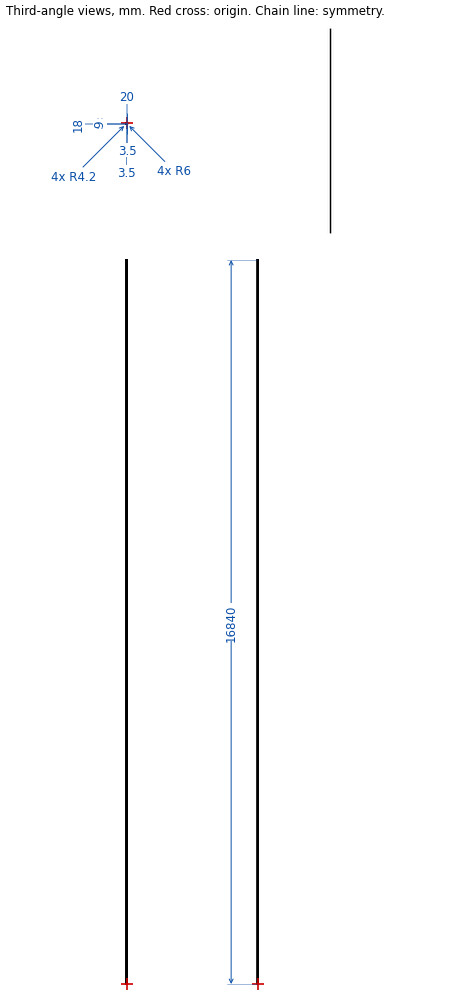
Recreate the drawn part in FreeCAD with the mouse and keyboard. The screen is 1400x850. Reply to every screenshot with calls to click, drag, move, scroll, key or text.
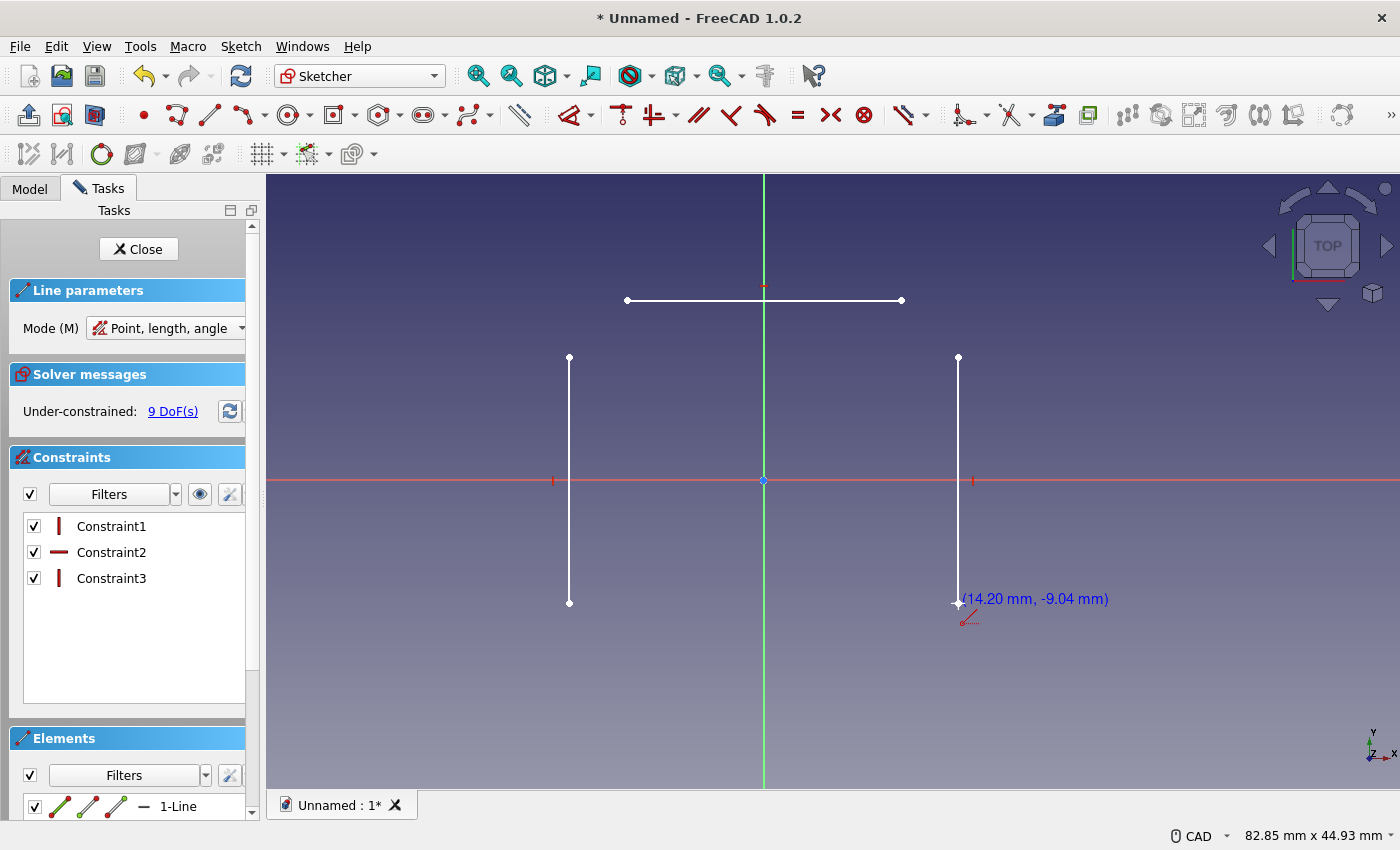
click(177, 116)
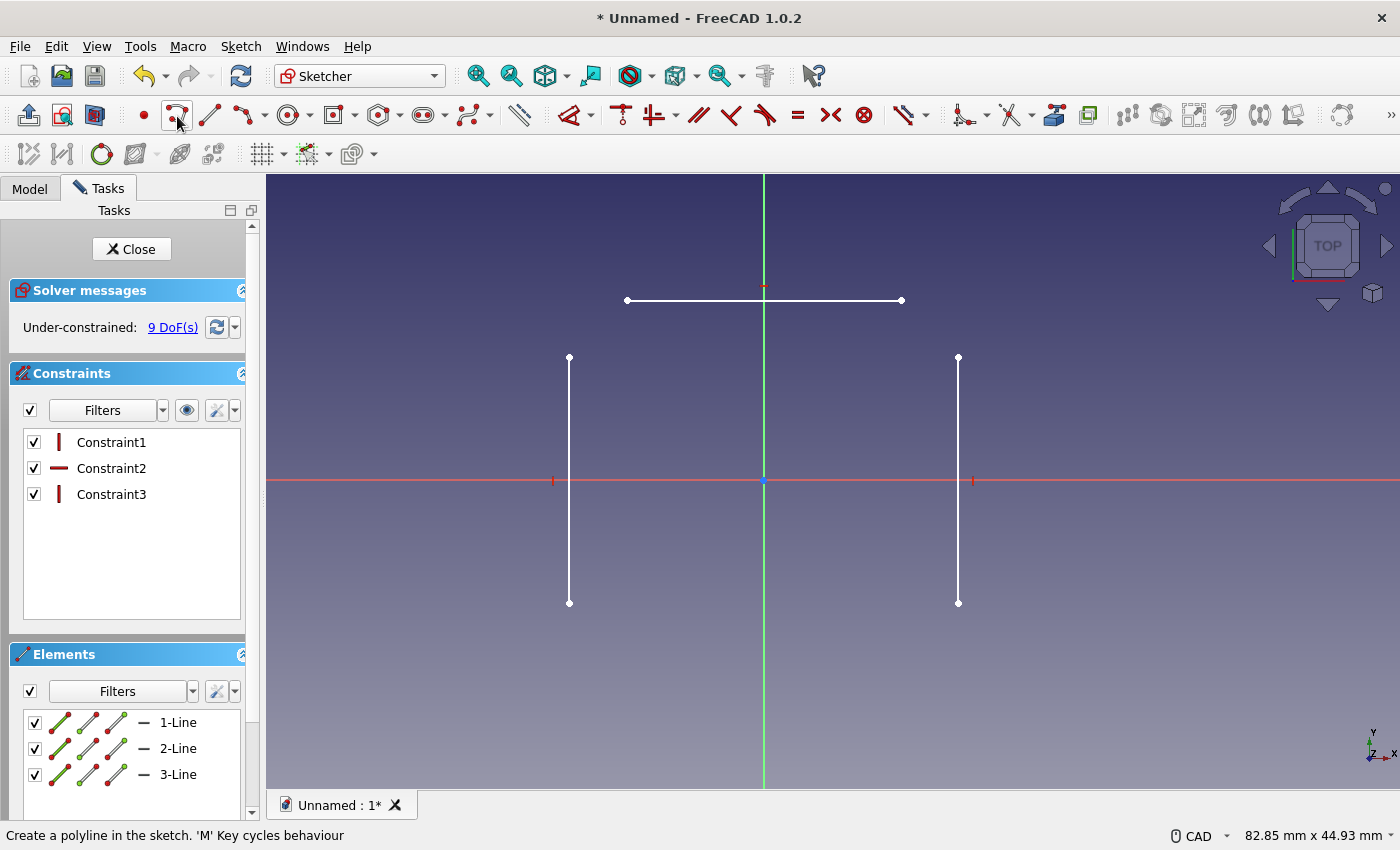
click(901, 661)
click(853, 661)
click(853, 686)
click(901, 686)
right_click(901, 686)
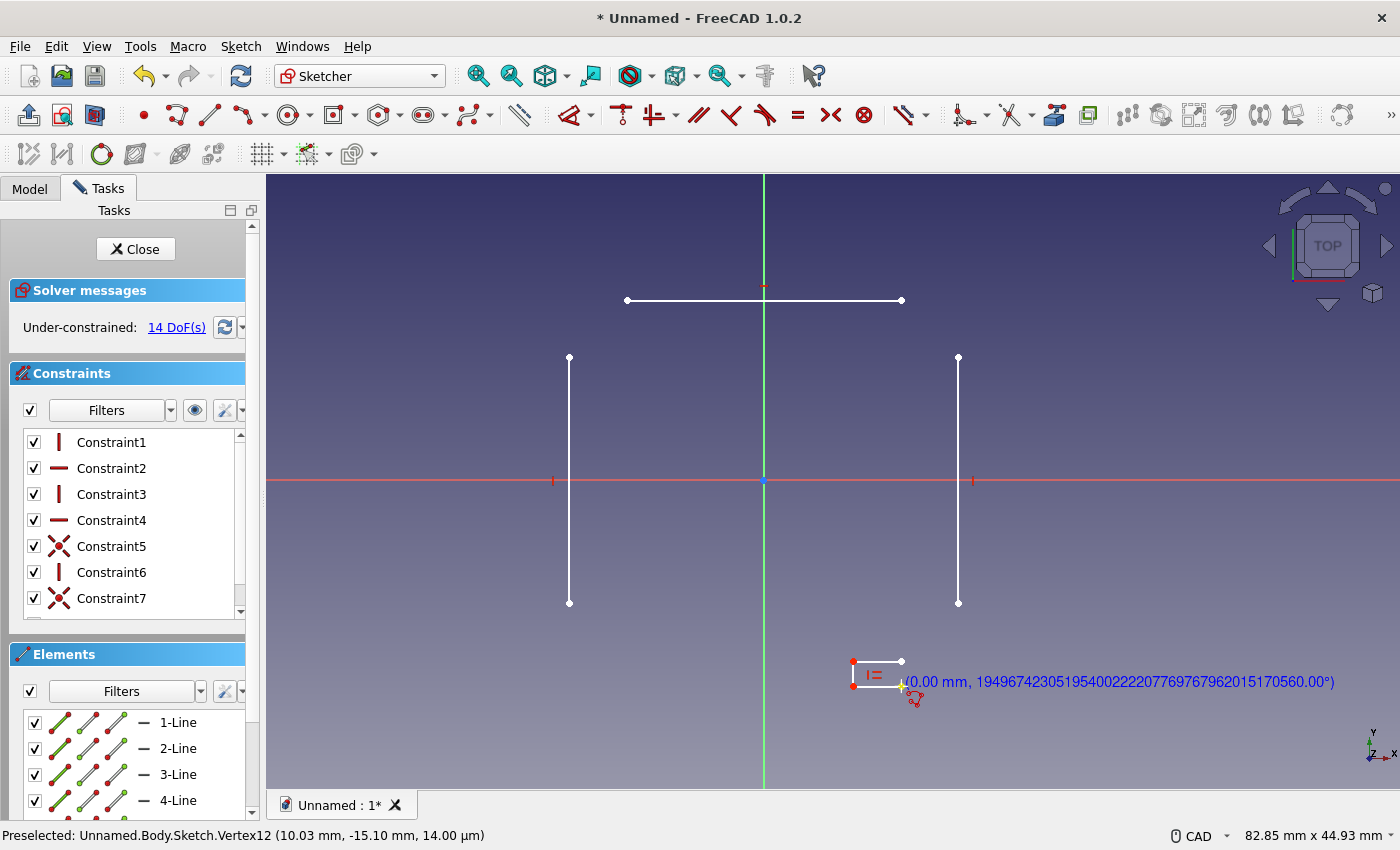
click(210, 116)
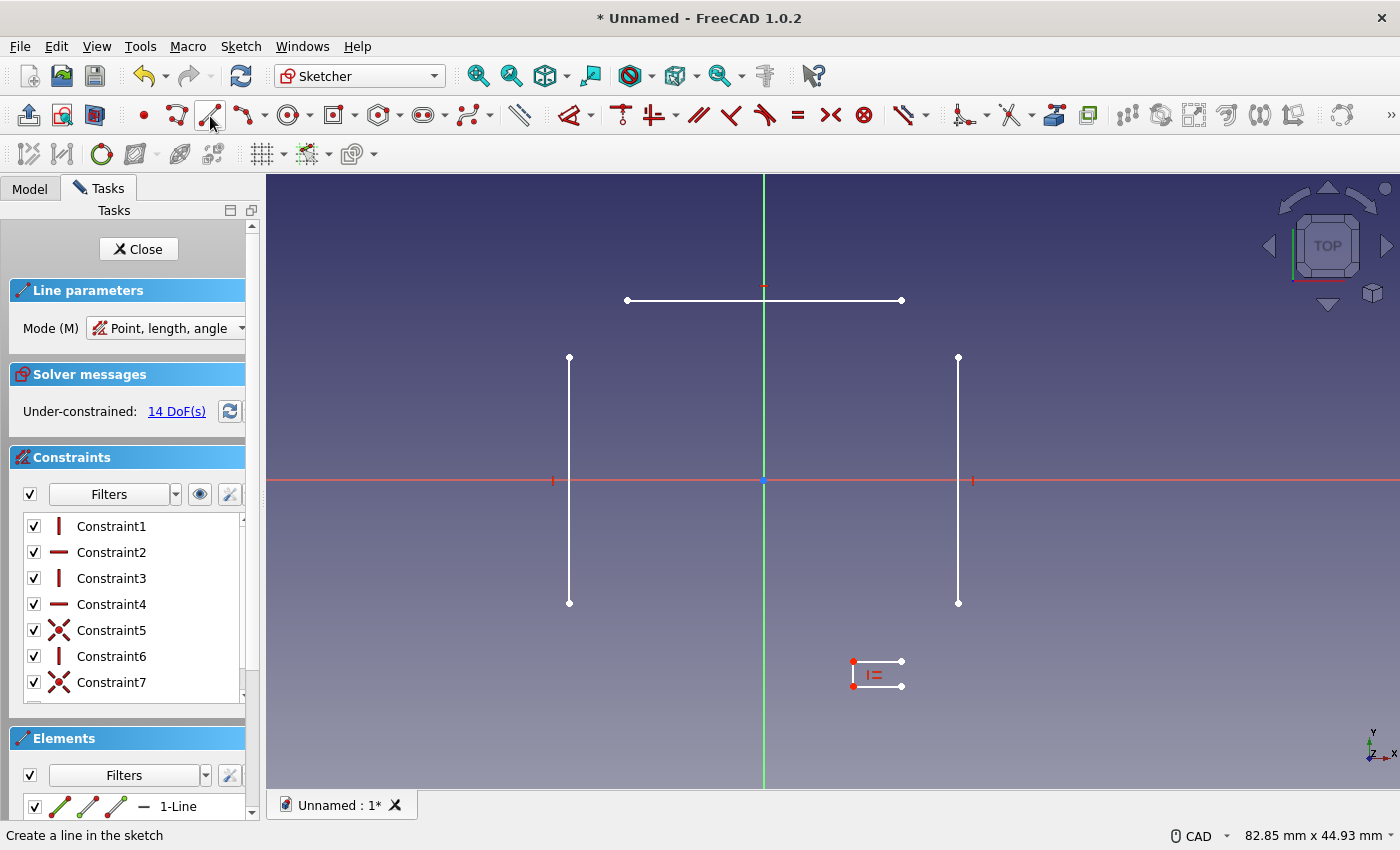
click(983, 603)
click(983, 357)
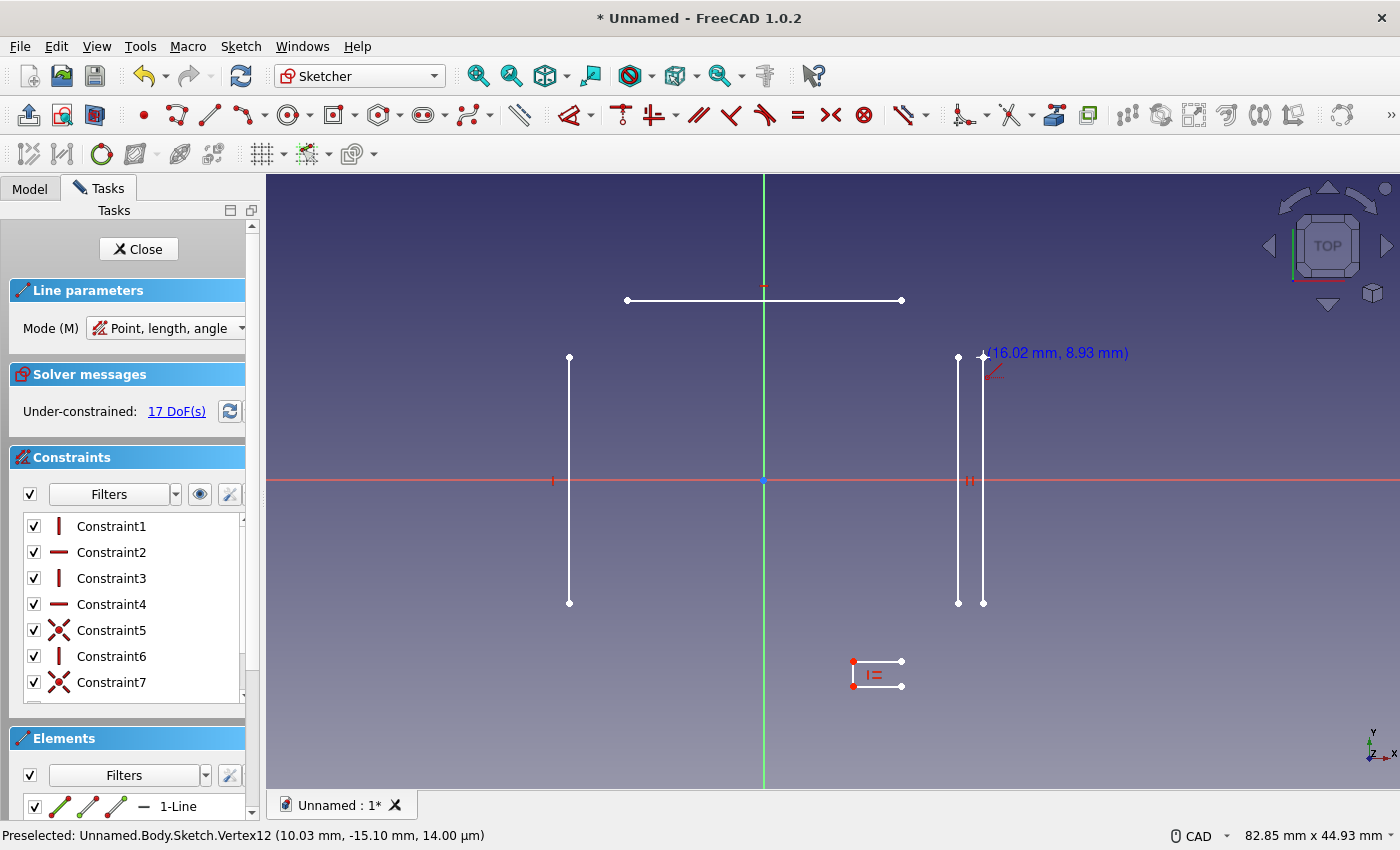
click(901, 275)
click(627, 275)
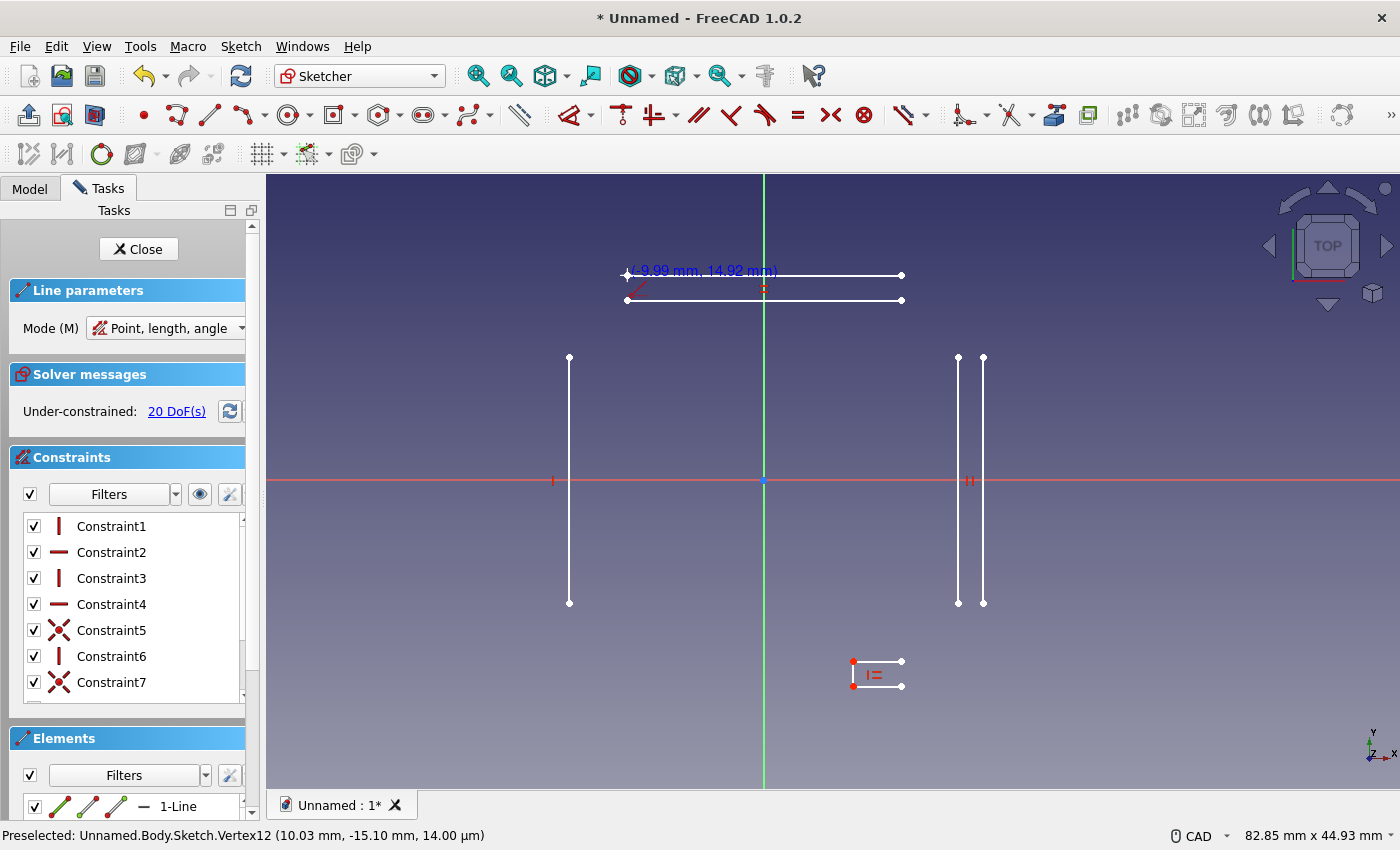
click(545, 357)
click(545, 603)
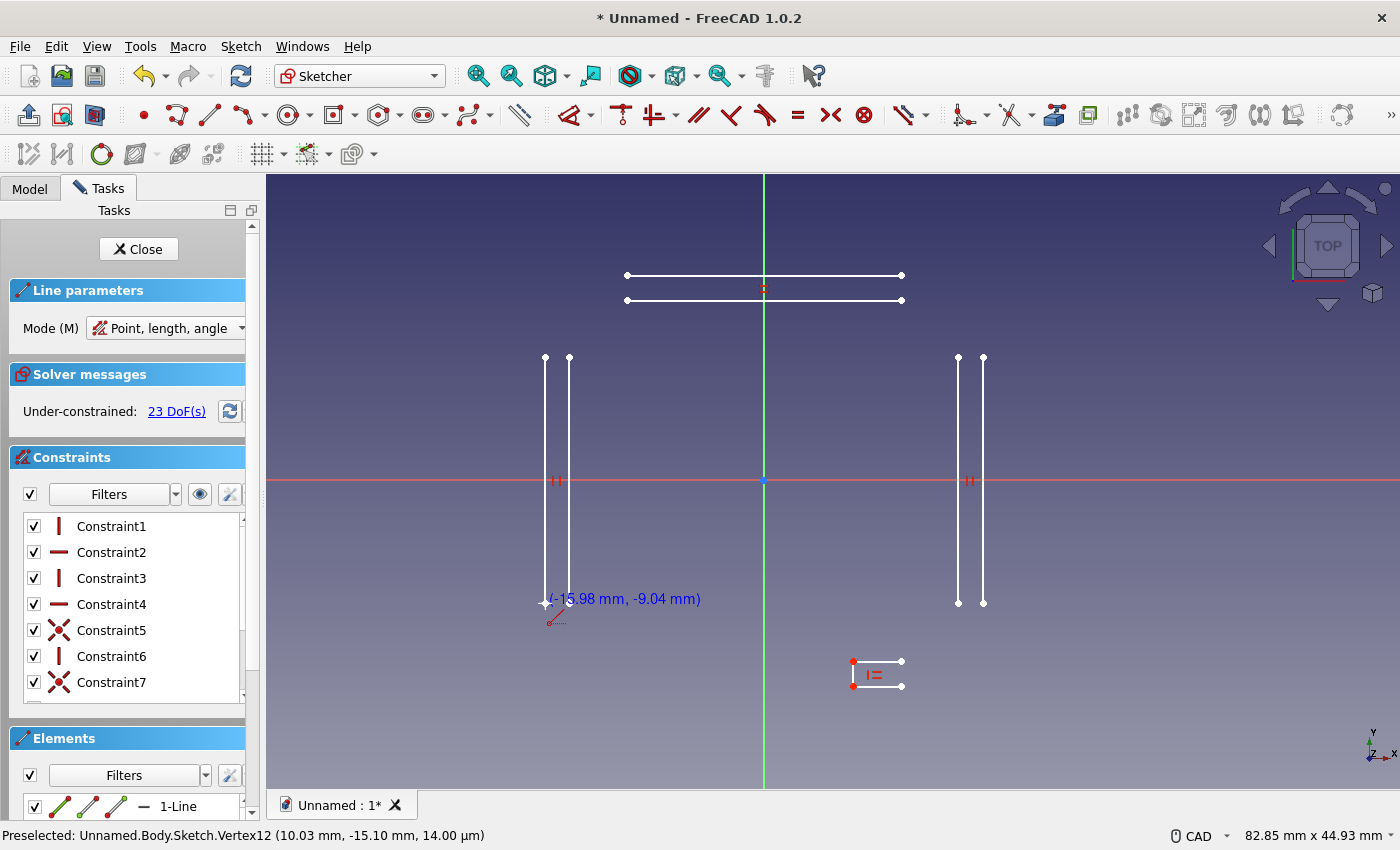
click(177, 116)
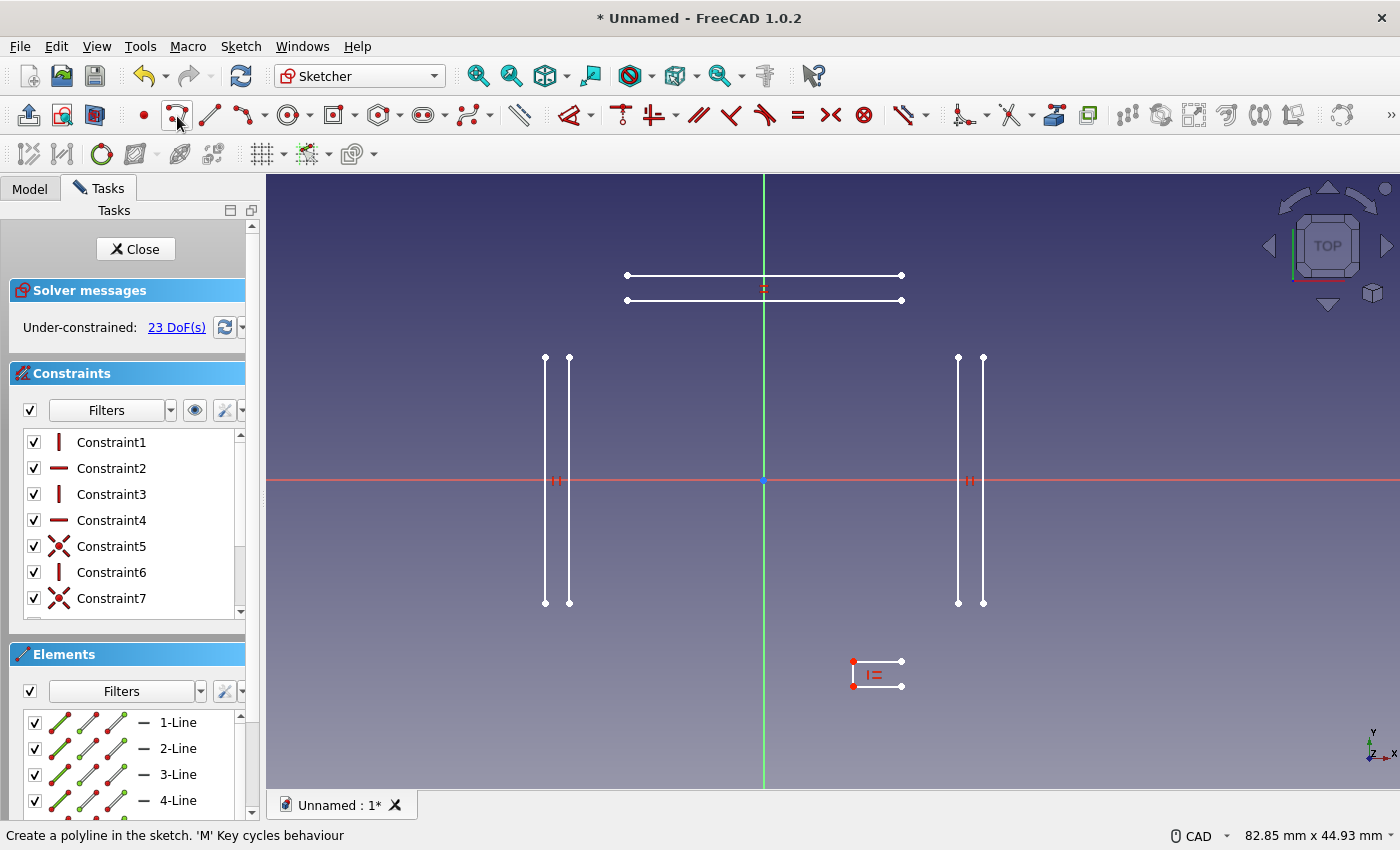
click(627, 686)
click(675, 686)
click(675, 661)
click(627, 661)
right_click(627, 661)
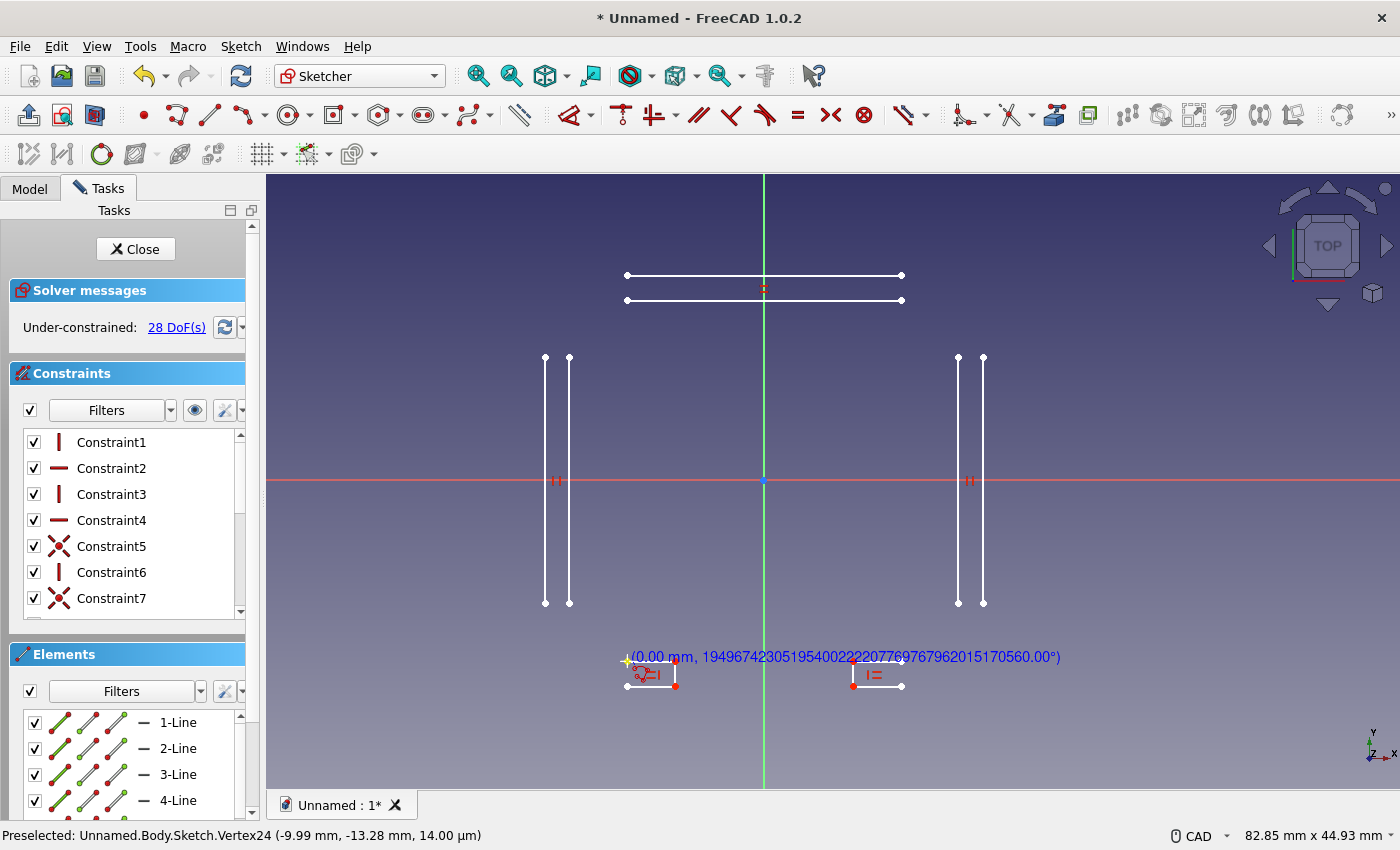
click(242, 116)